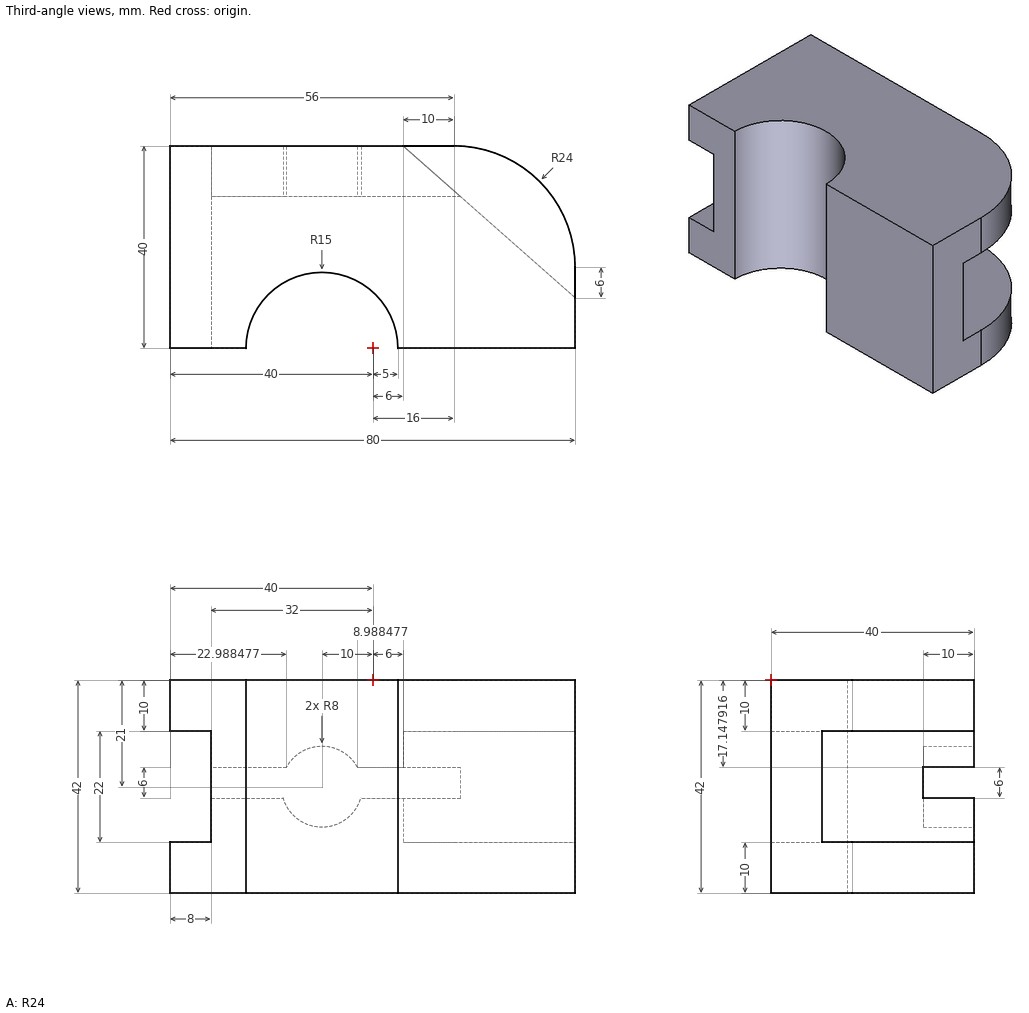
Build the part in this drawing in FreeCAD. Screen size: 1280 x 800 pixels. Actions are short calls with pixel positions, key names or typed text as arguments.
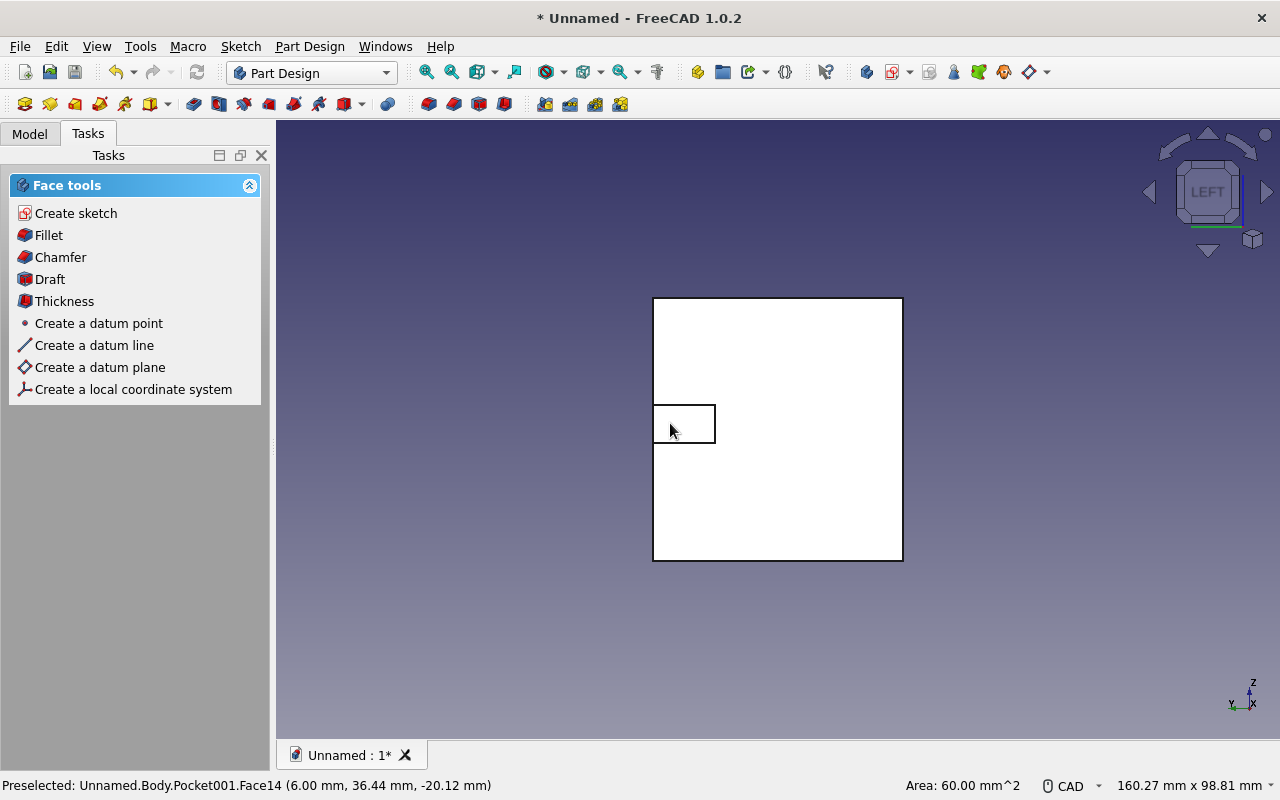
click(892, 72)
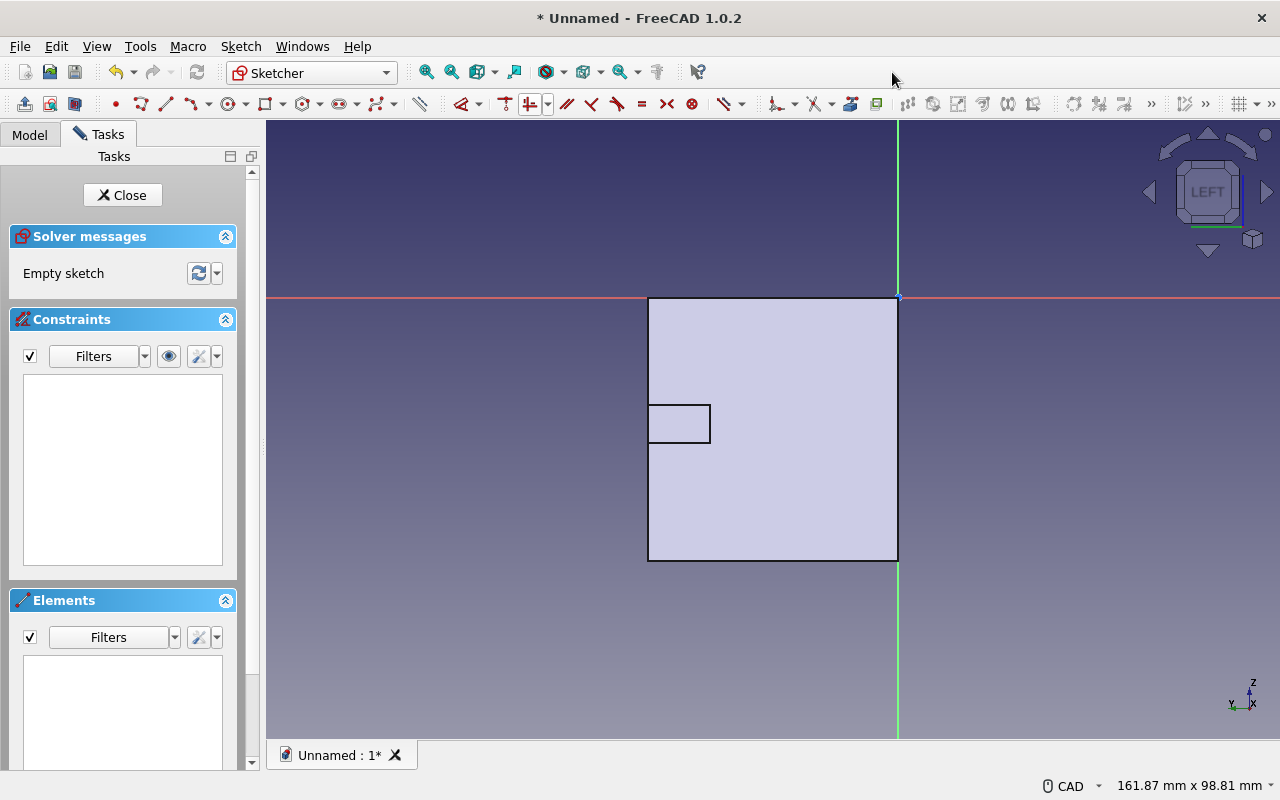
key(q)
key(s)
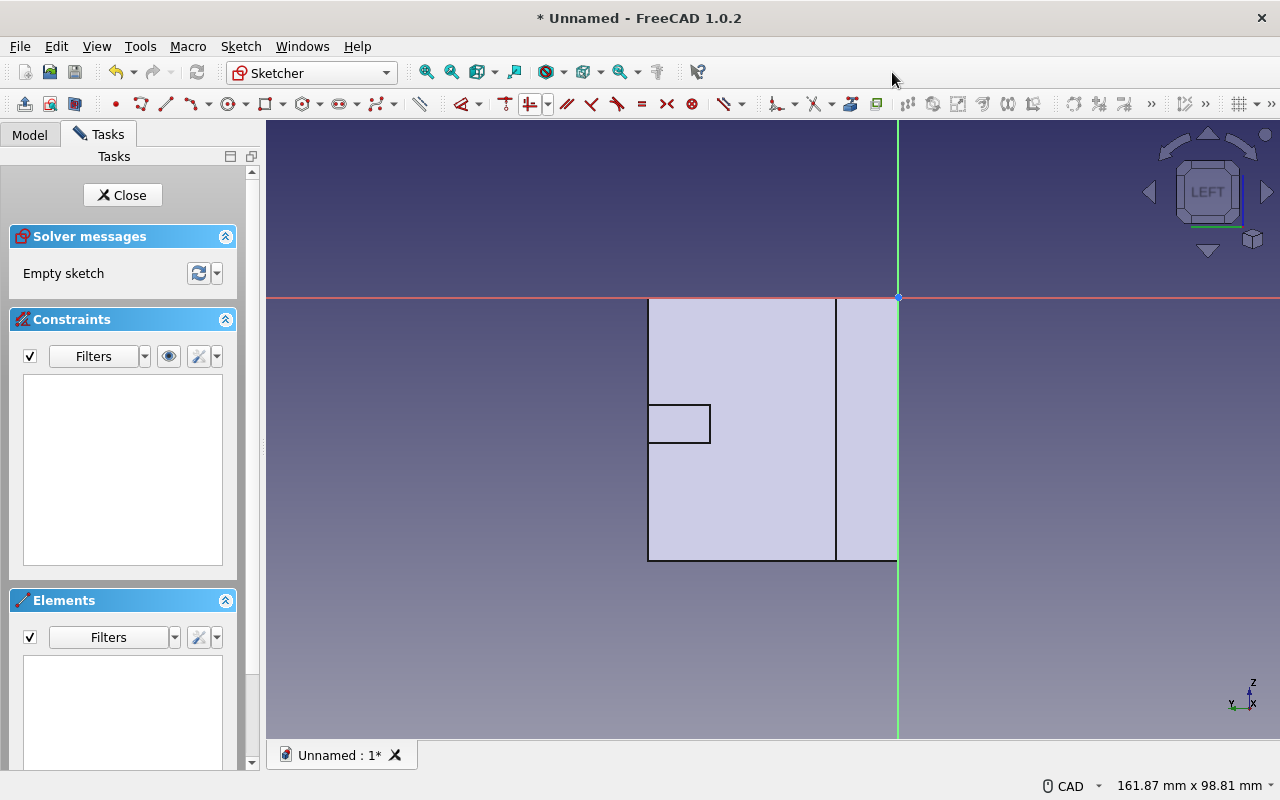
scroll(676, 423, up, 11)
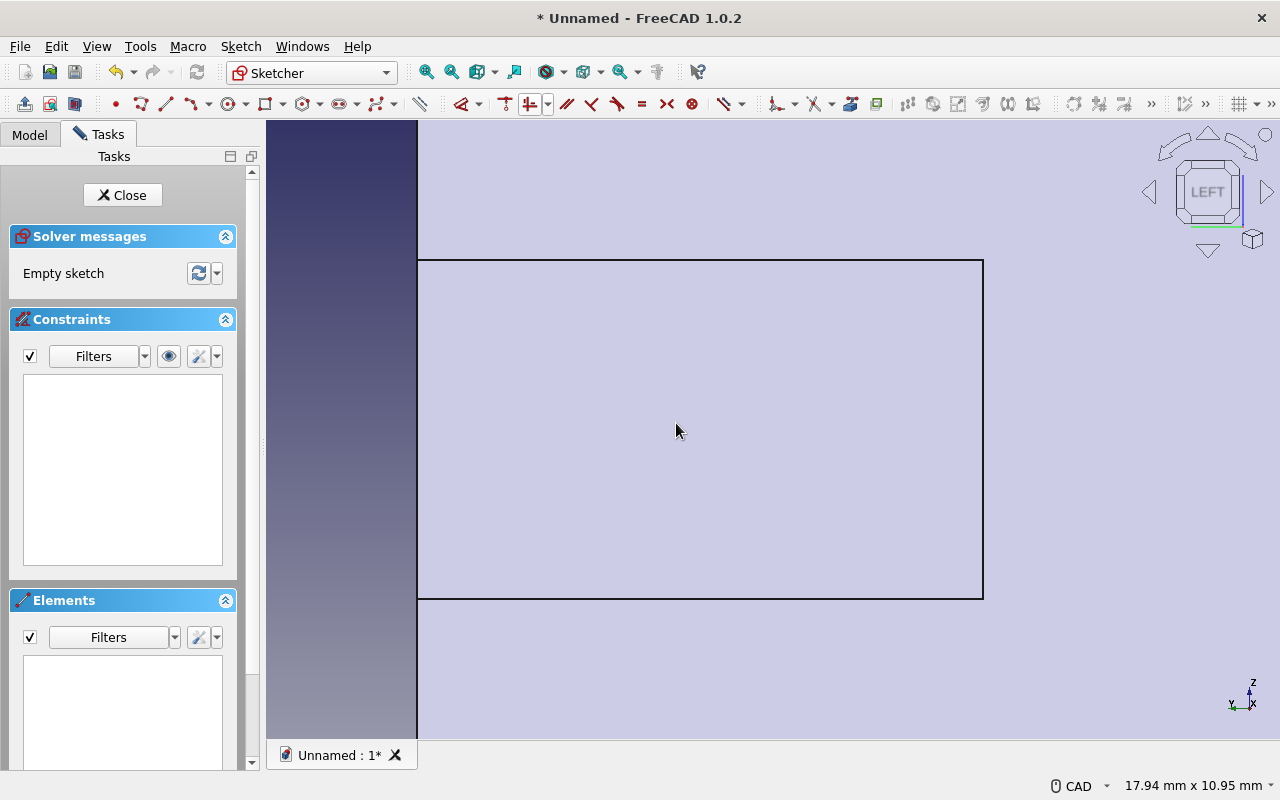
key(g)
key(r)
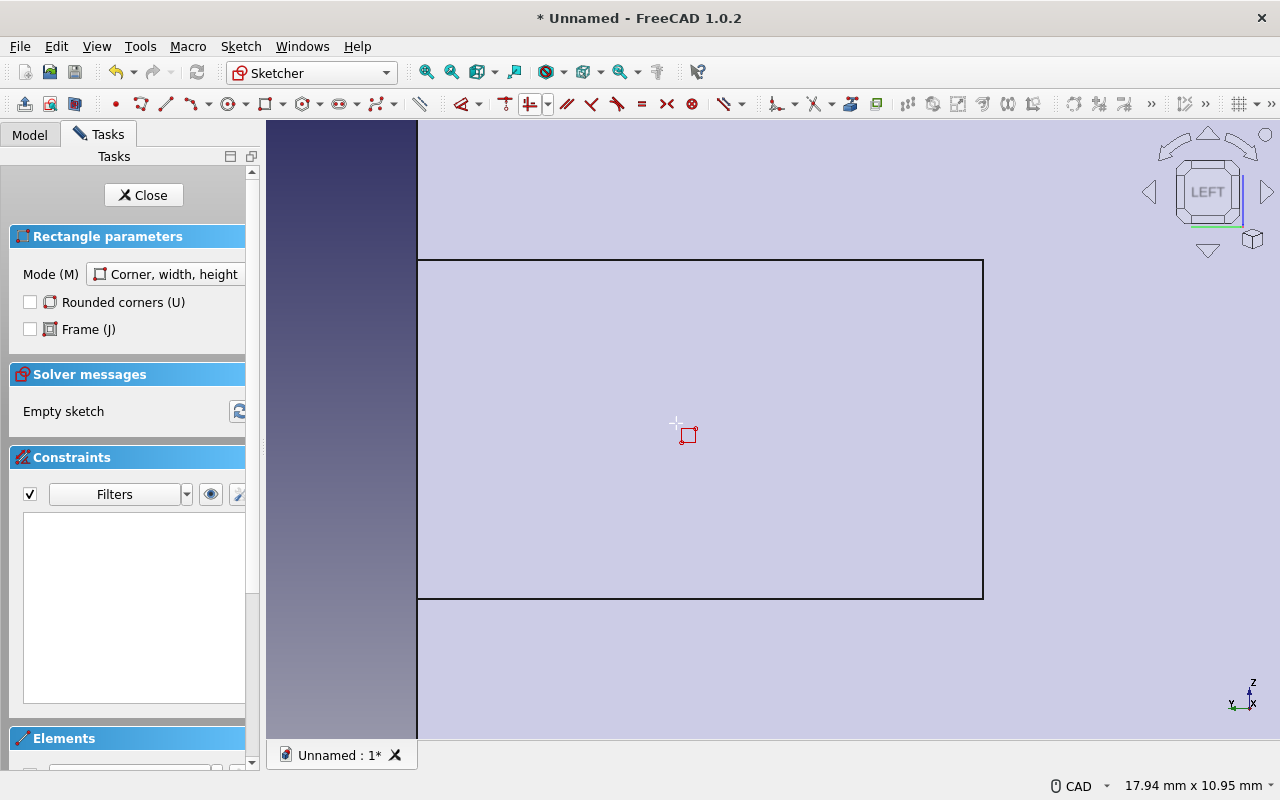
click(417, 260)
move(983, 599)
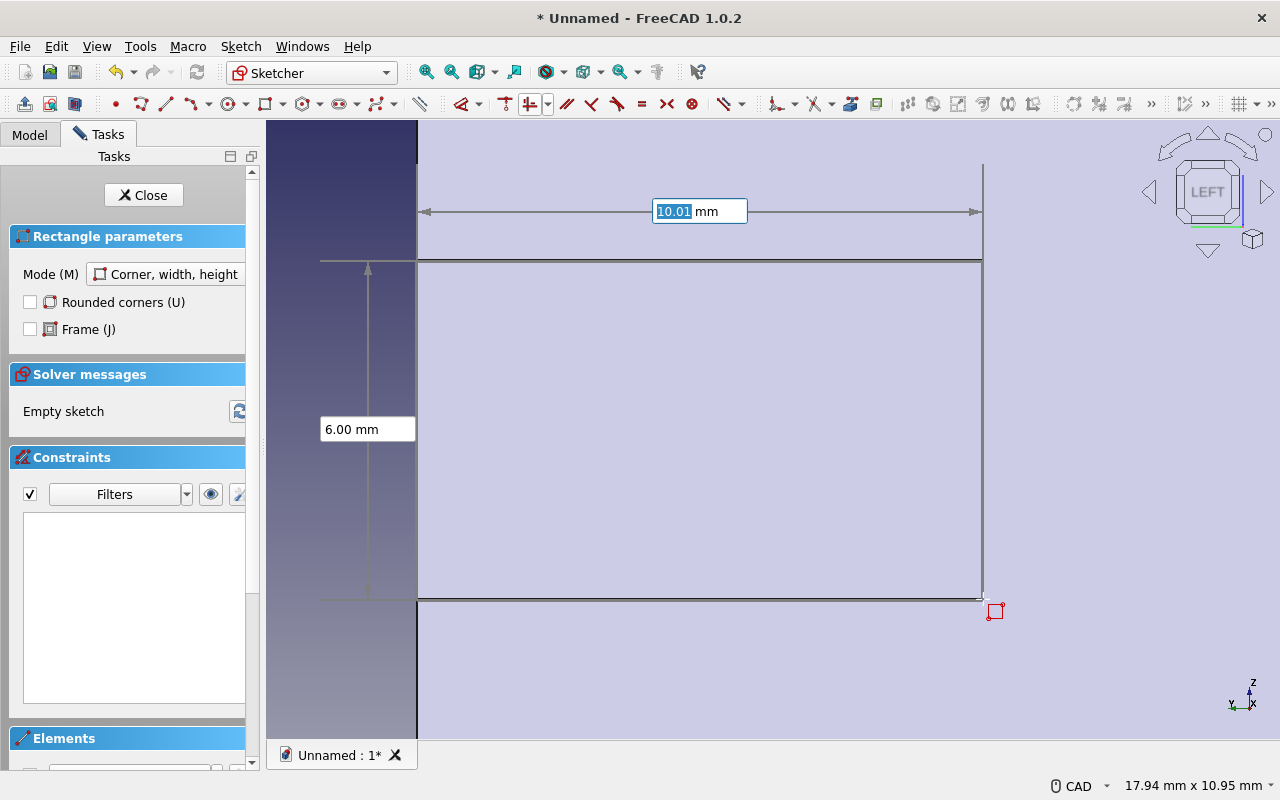
text(10)
key(Tab)
text(6)
key(Return)
key(Escape)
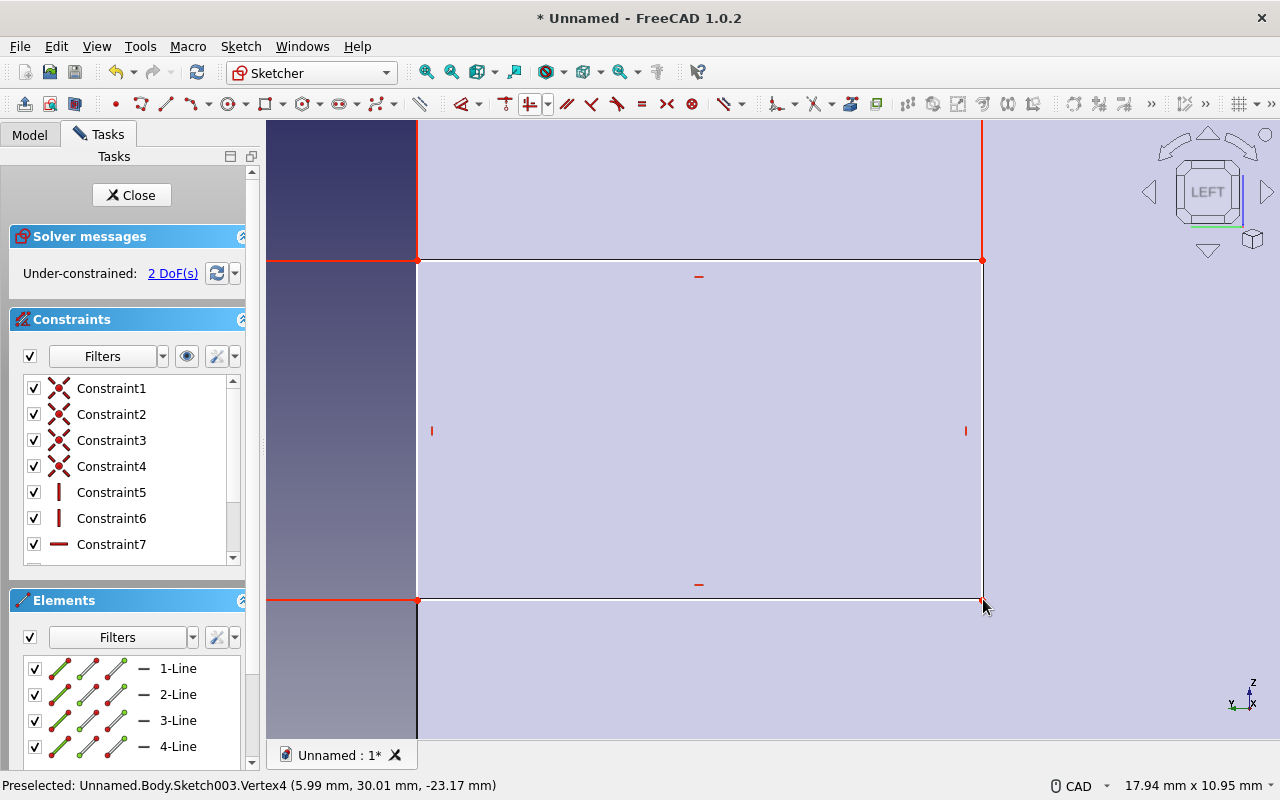
key(d)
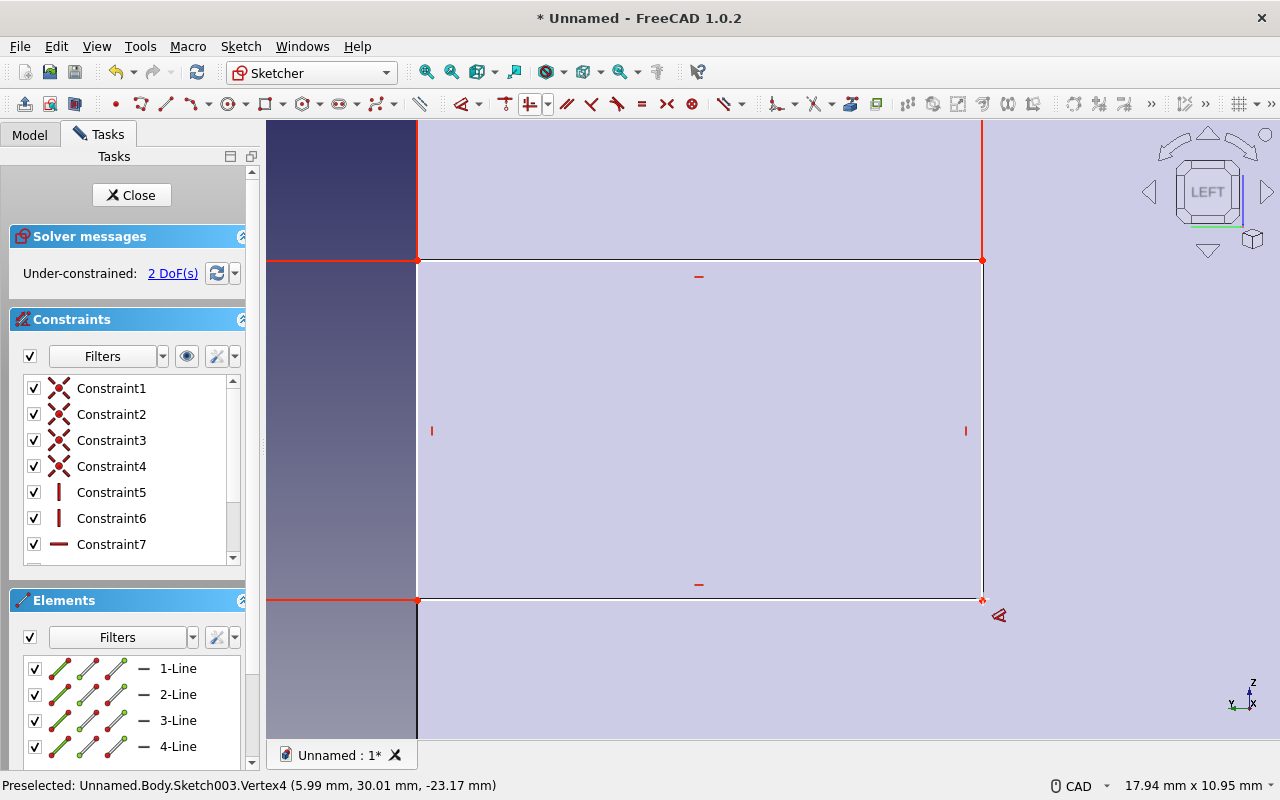
click(417, 261)
click(766, 295)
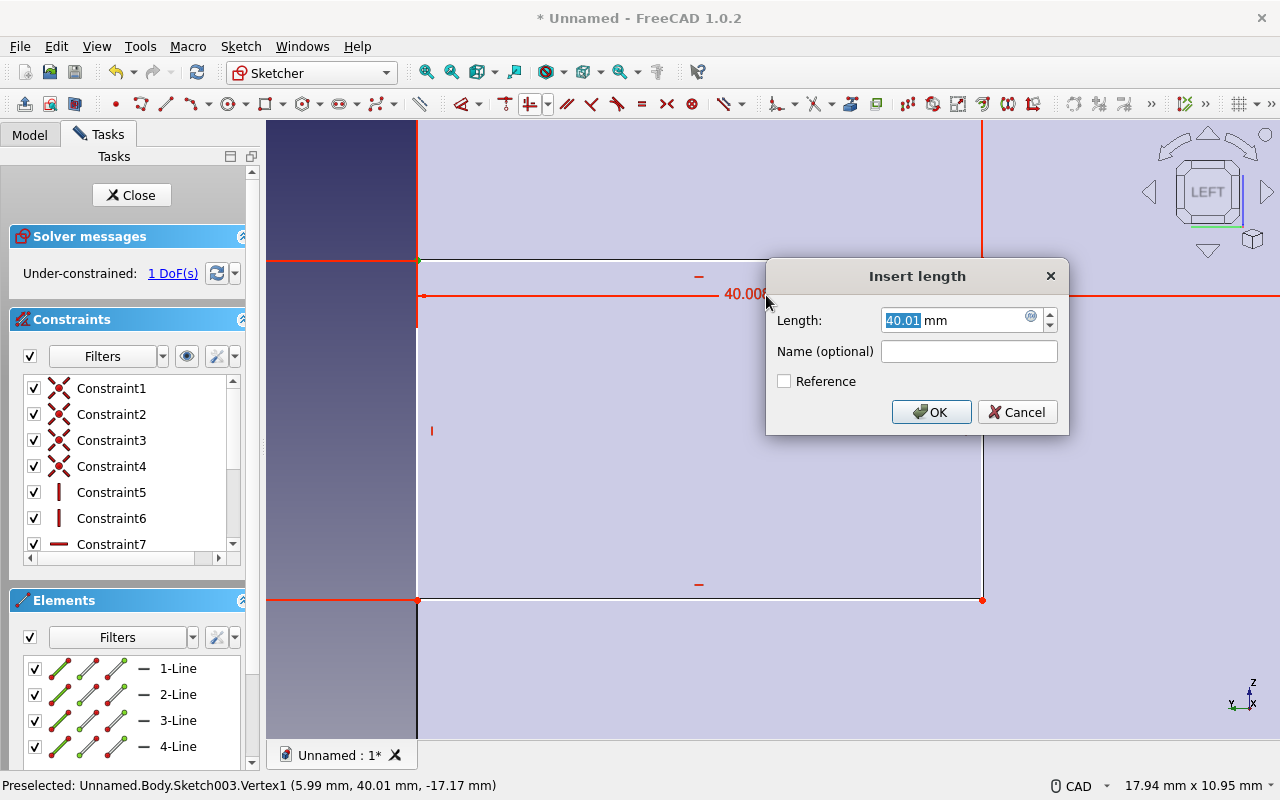
text(40)
key(Return)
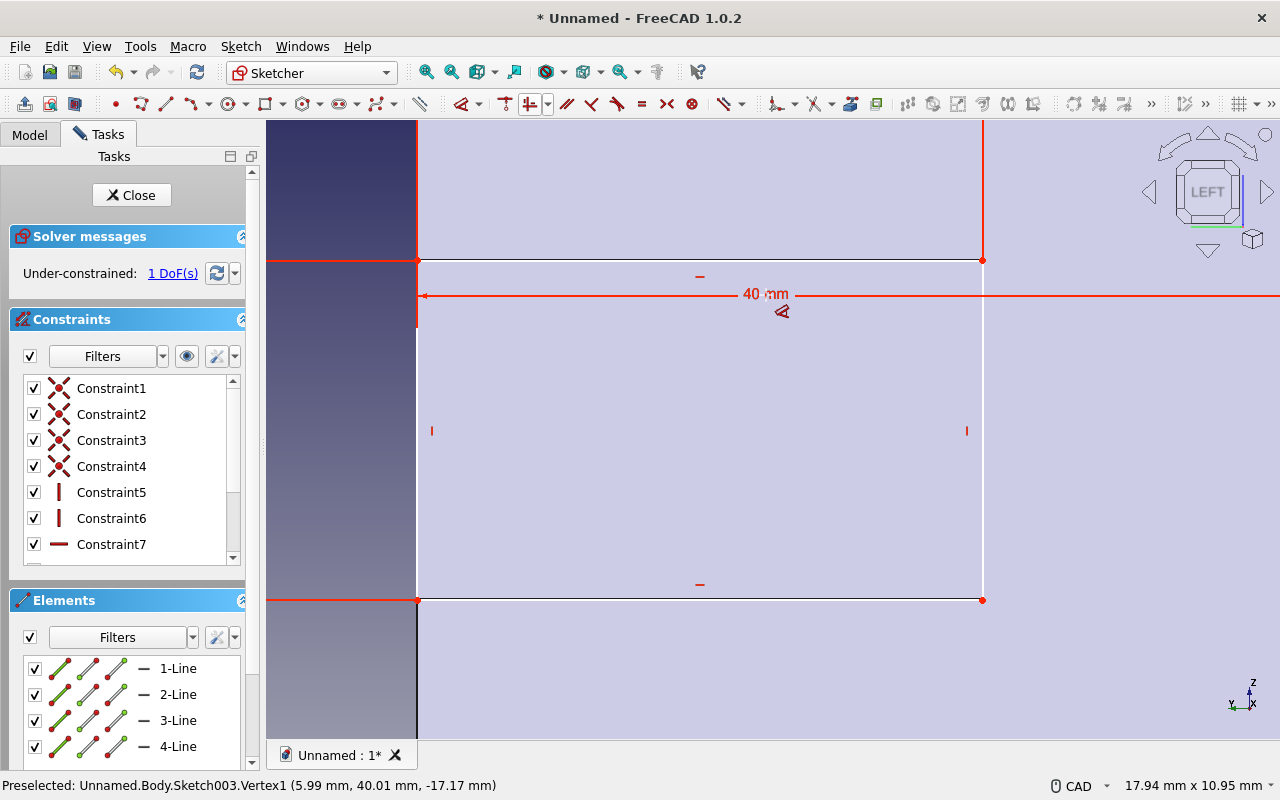
click(417, 261)
click(383, 204)